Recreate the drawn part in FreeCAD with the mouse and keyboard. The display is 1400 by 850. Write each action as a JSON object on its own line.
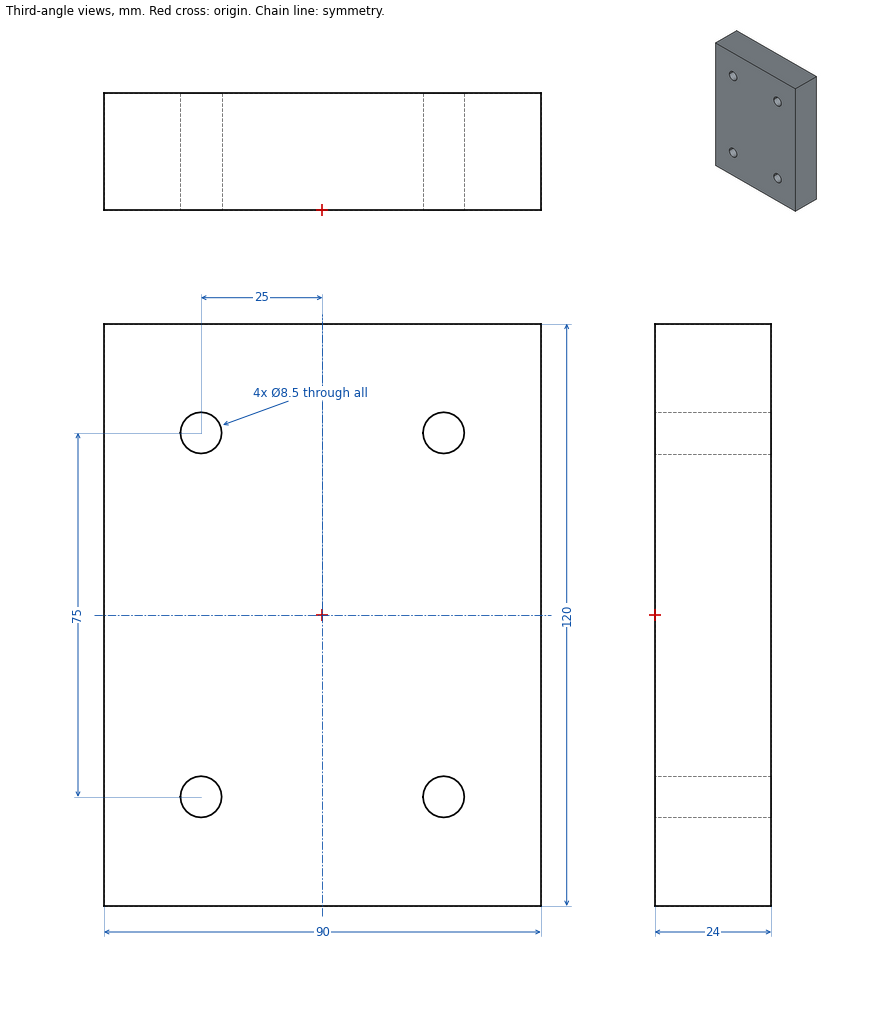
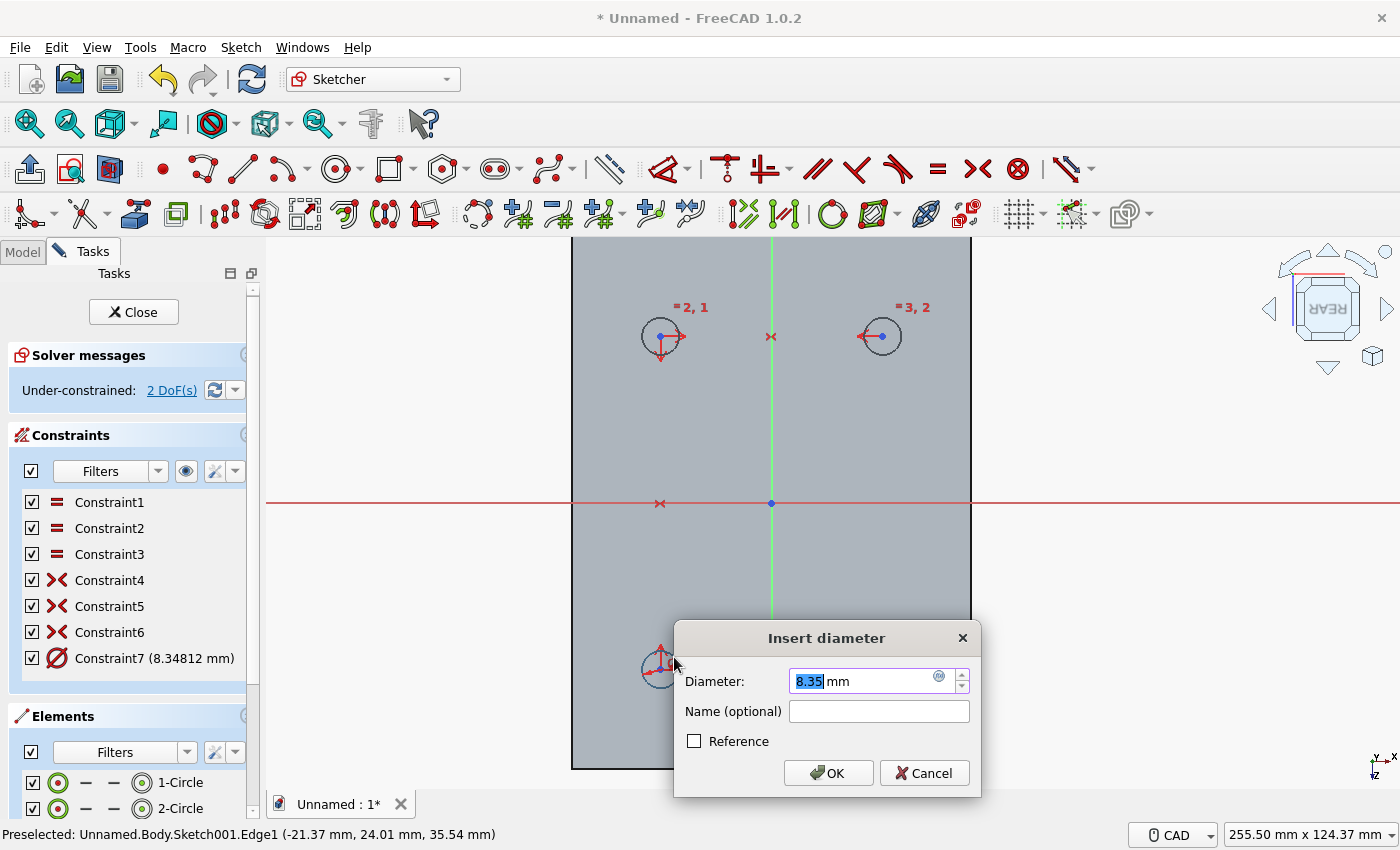
{"action": "type", "text": "8.5"}
{"action": "key", "text": "Return"}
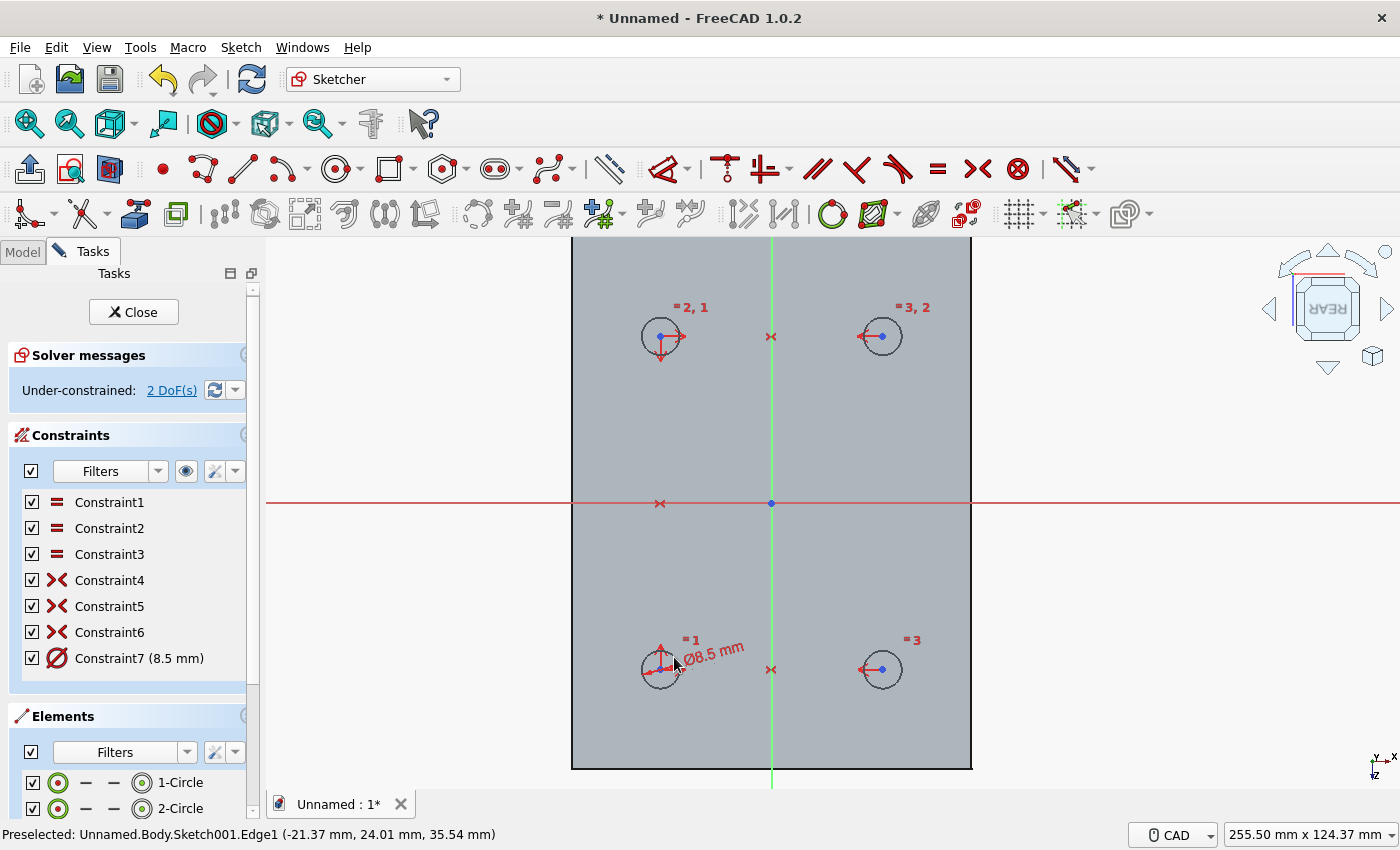
{"action": "left_click", "coordinate": [661, 670]}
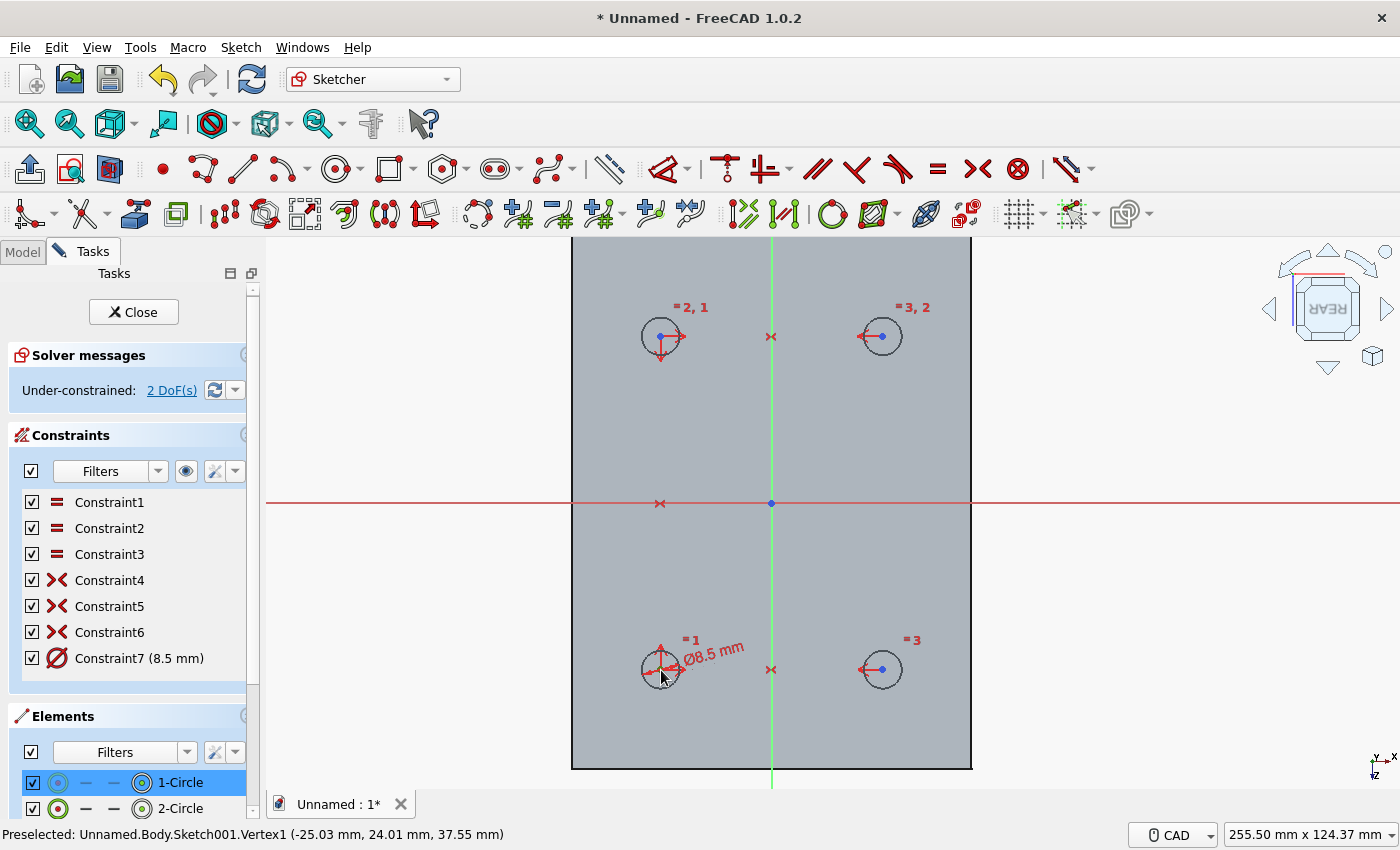
{"action": "key", "text": "l"}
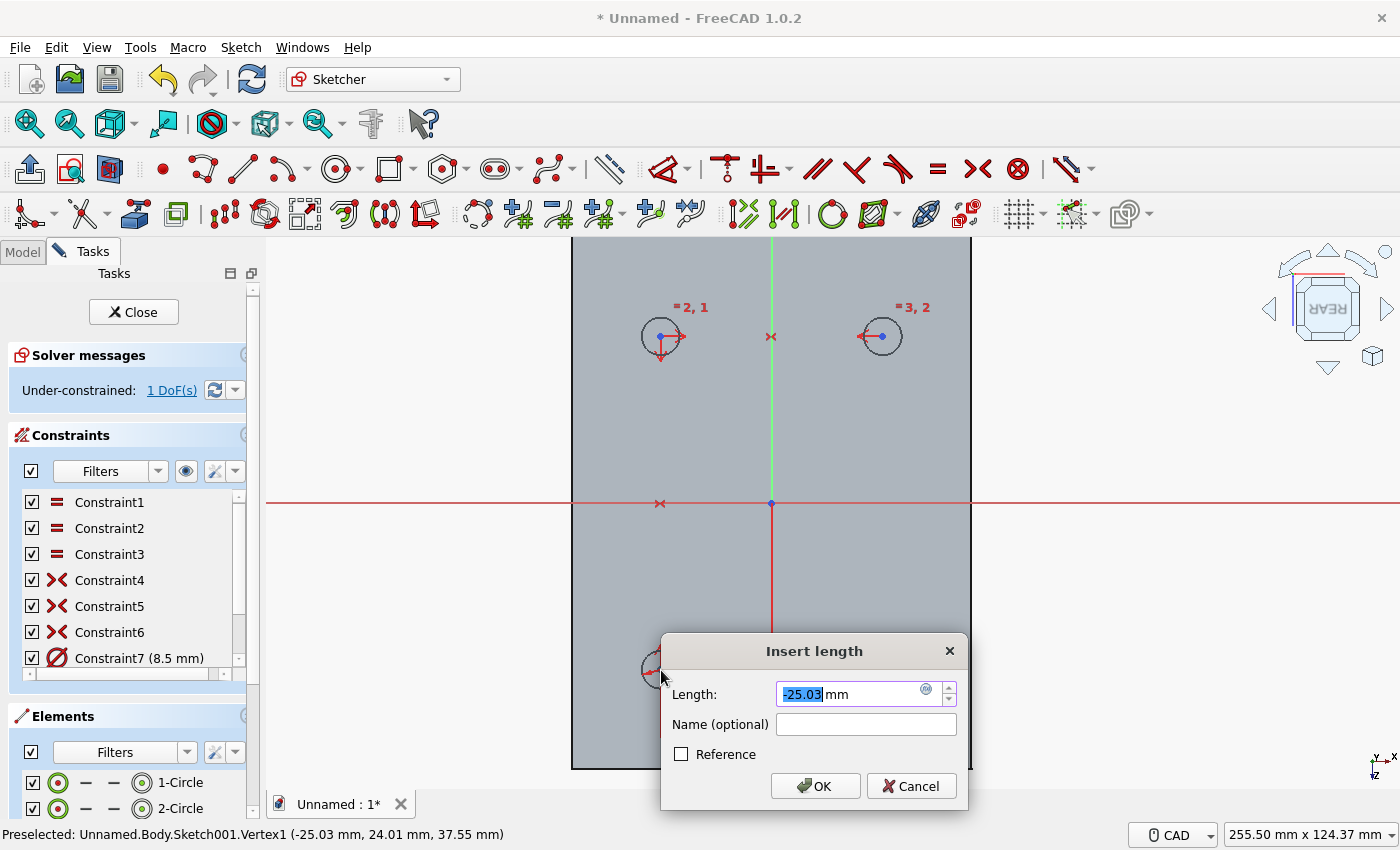
{"action": "type", "text": "-25"}
{"action": "key", "text": "Return"}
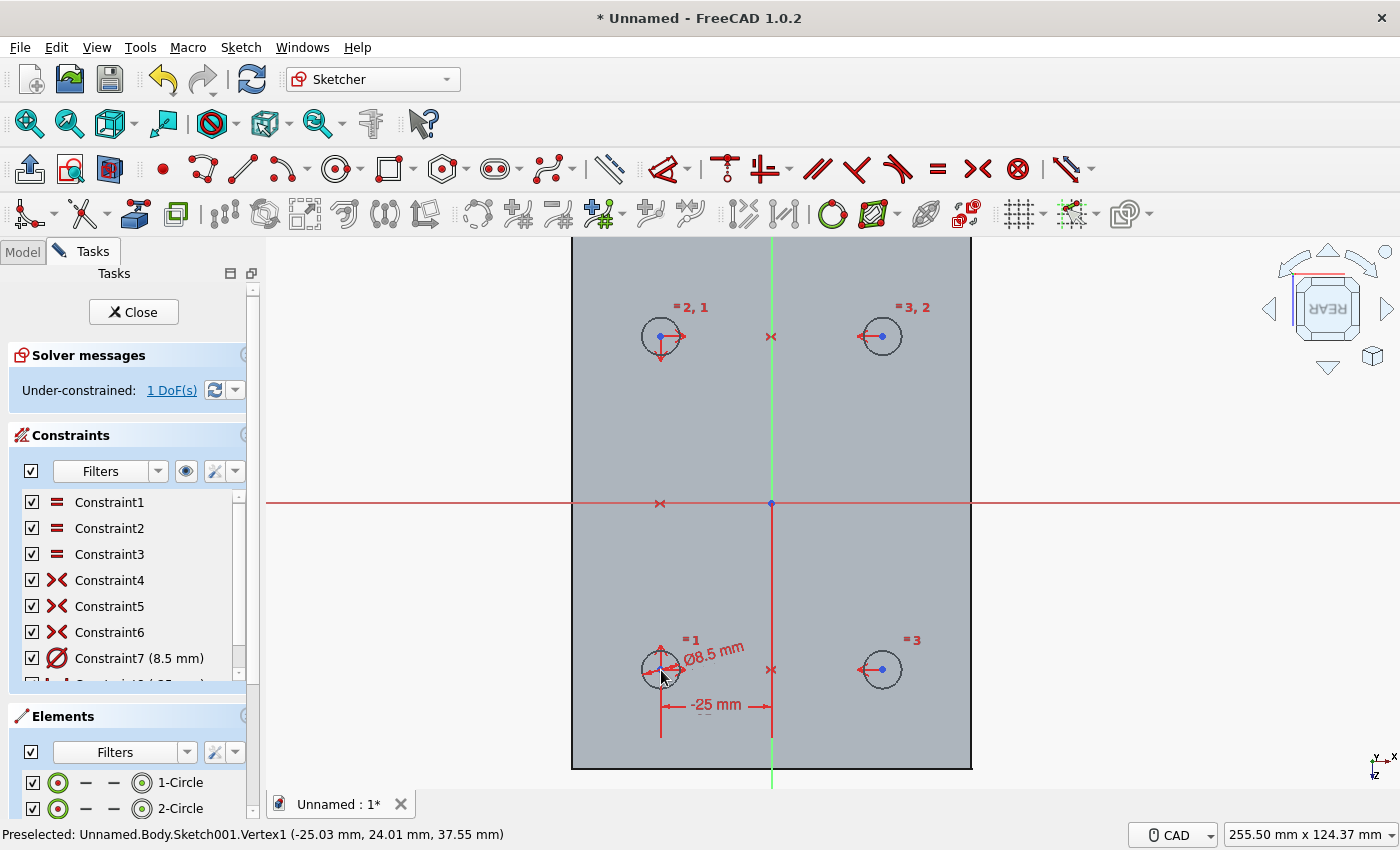
{"action": "left_click", "coordinate": [661, 670]}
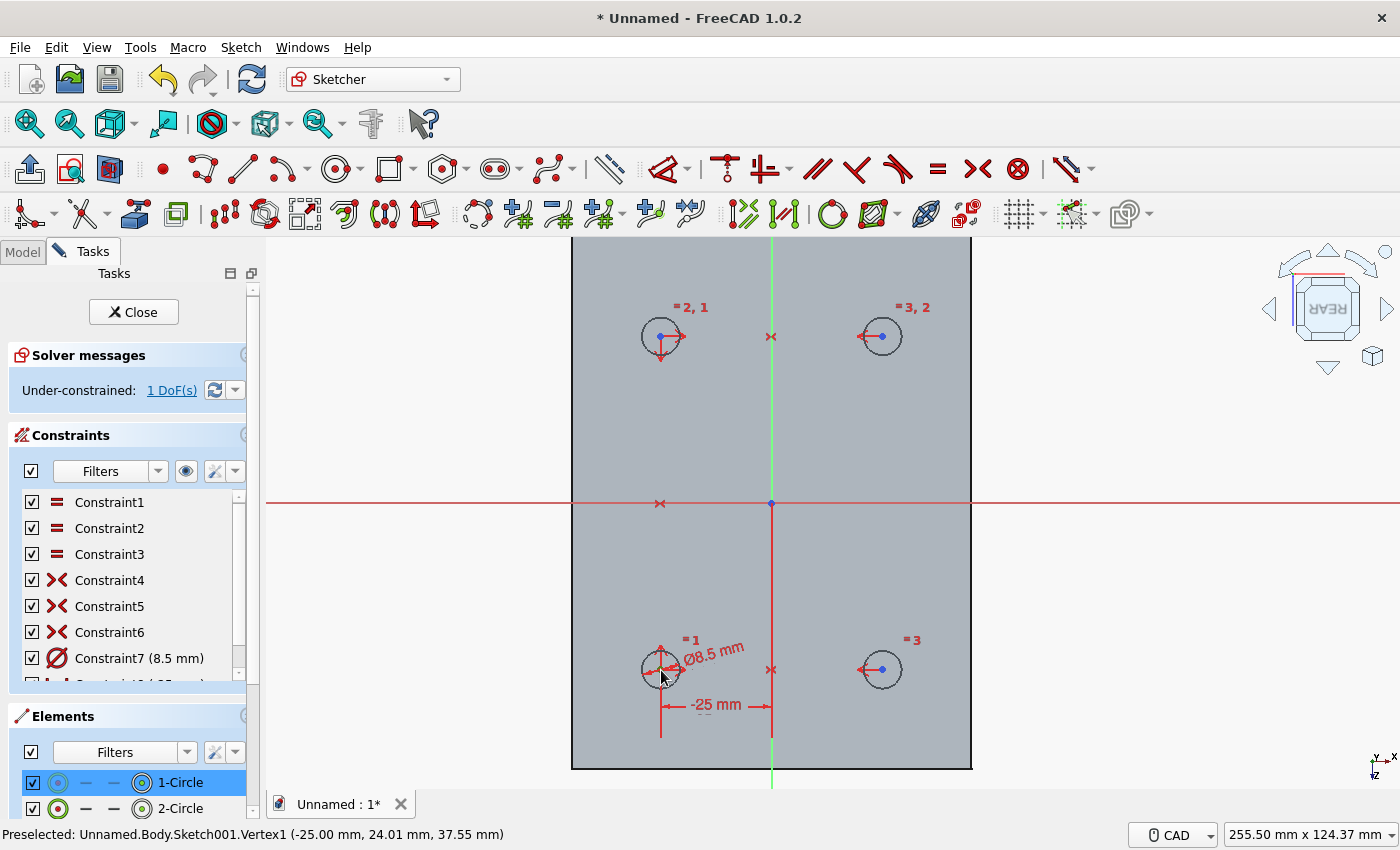
{"action": "left_click", "coordinate": [661, 336]}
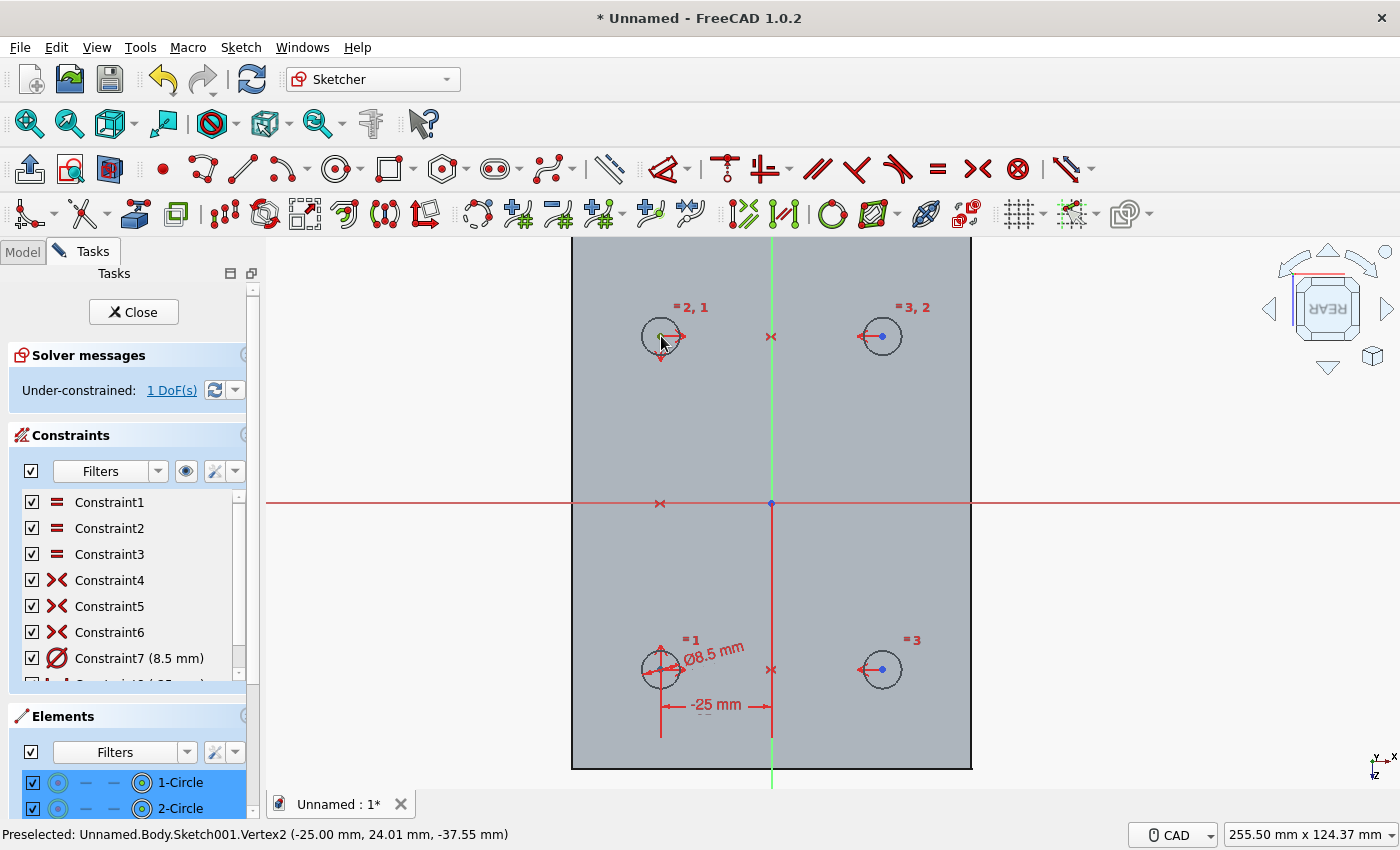
{"action": "left_click", "coordinate": [690, 170]}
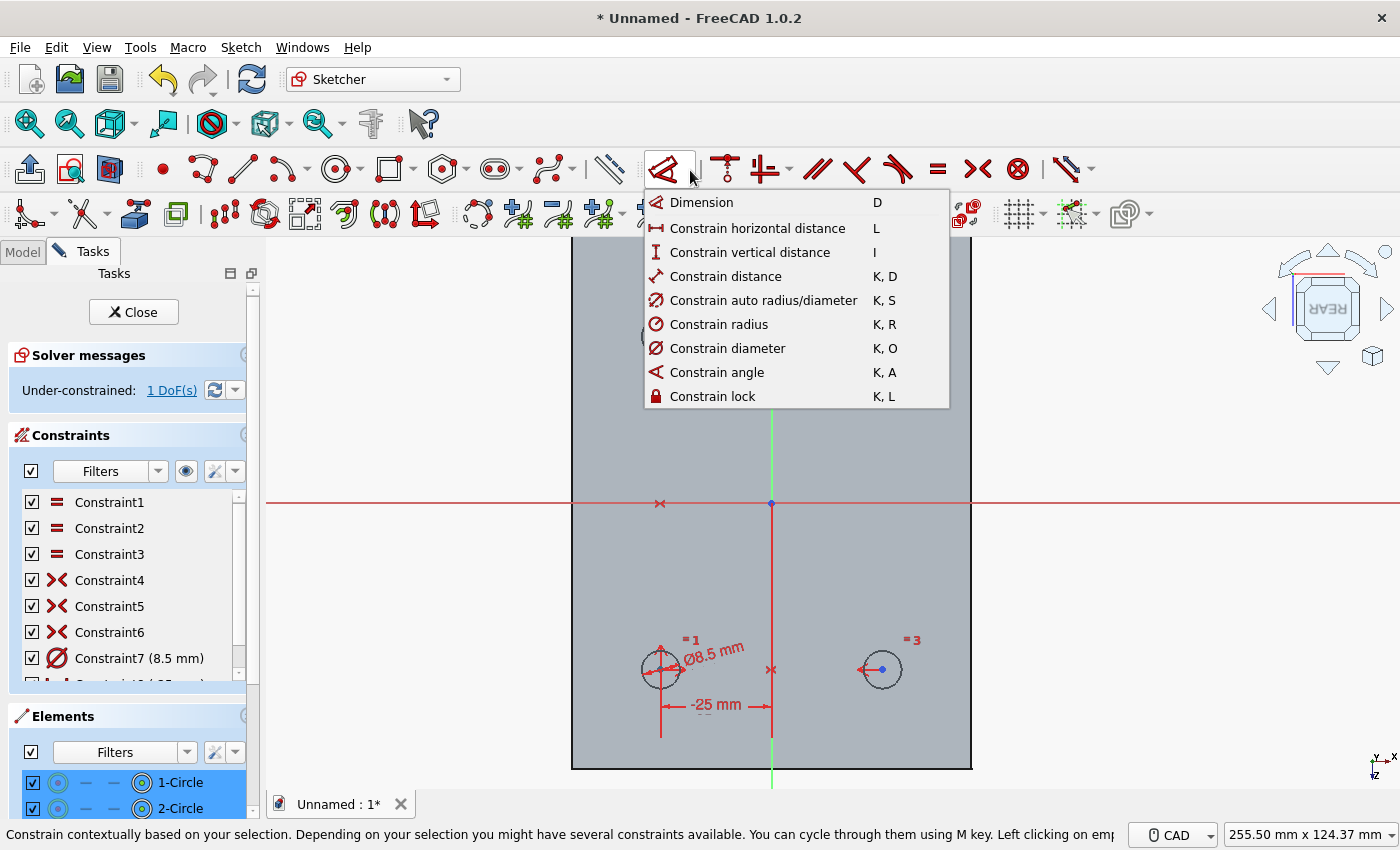
{"action": "left_click", "coordinate": [797, 252]}